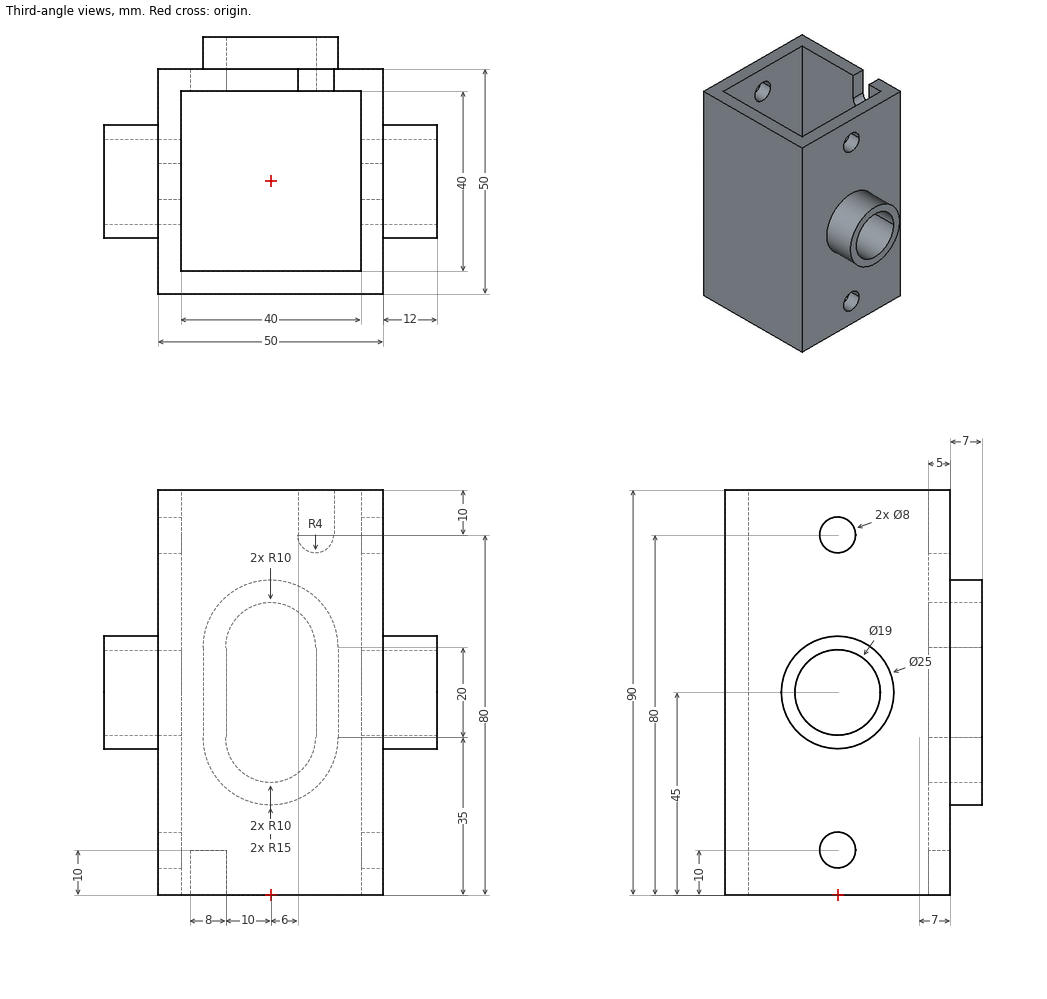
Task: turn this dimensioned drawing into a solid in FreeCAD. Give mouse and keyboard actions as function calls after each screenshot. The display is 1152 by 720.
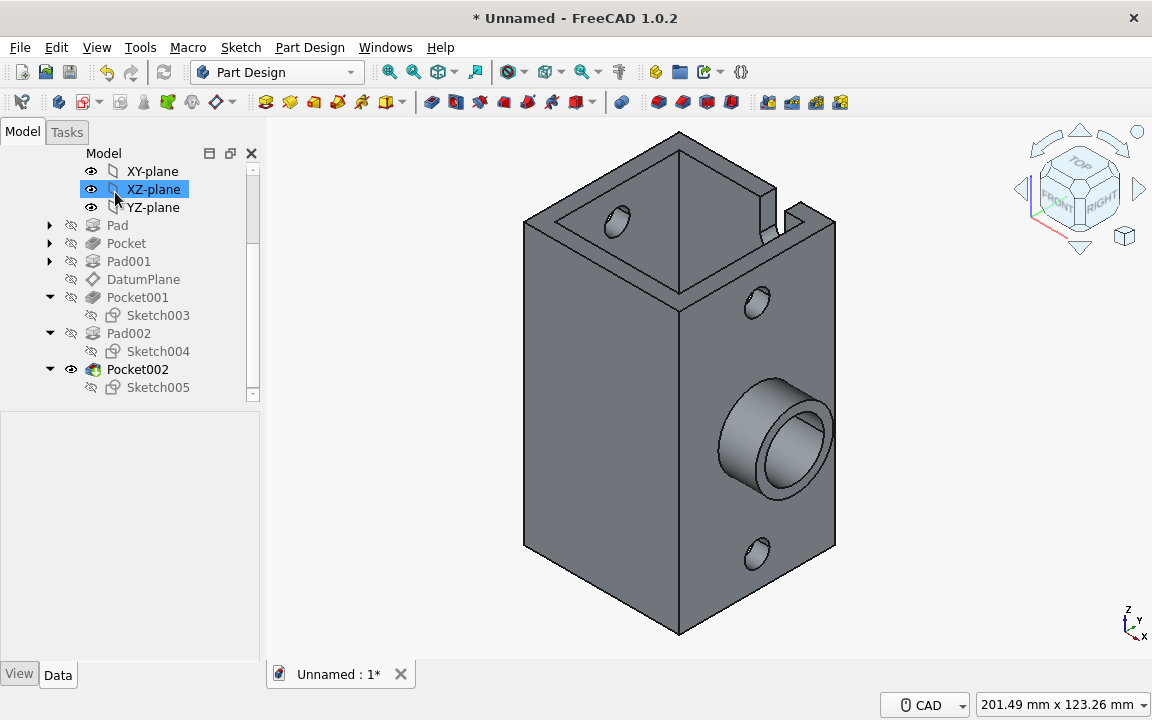
click(116, 333)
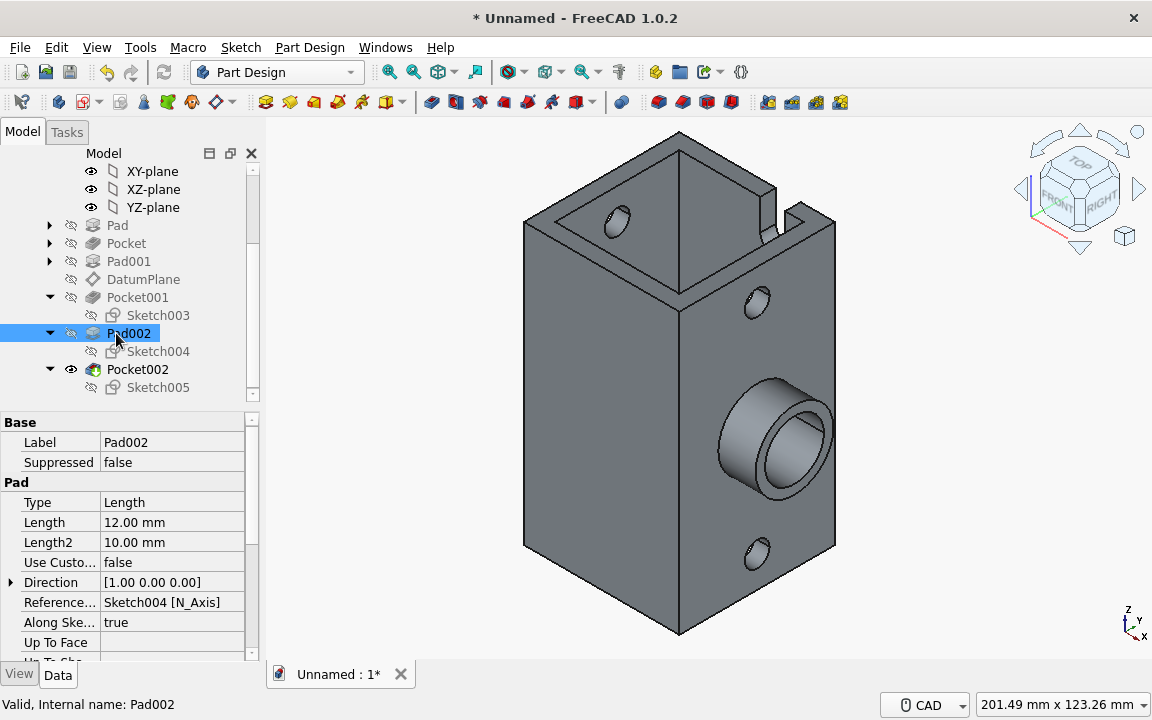
click(768, 102)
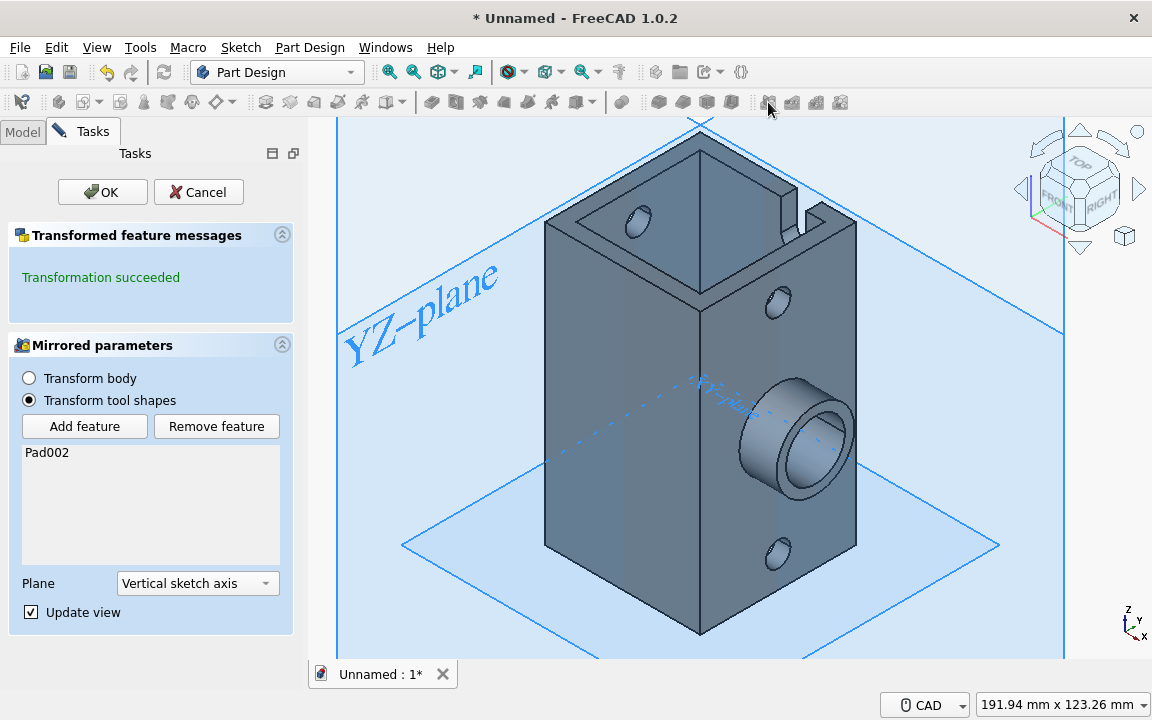
click(198, 584)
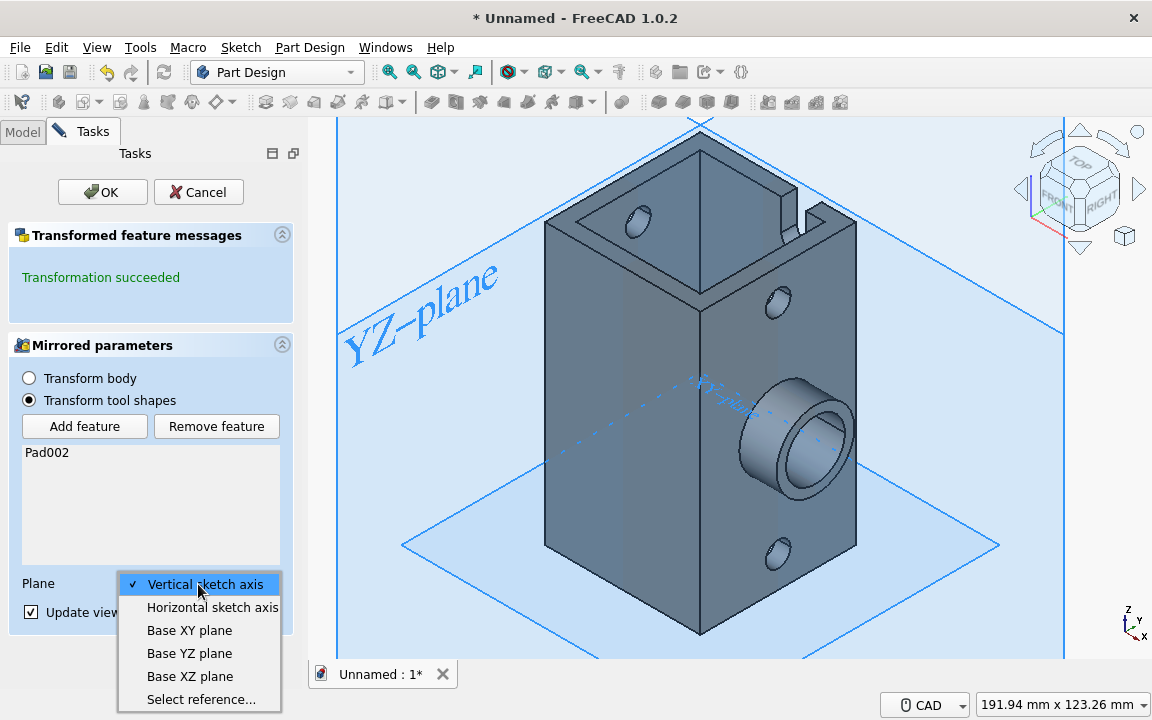
click(198, 654)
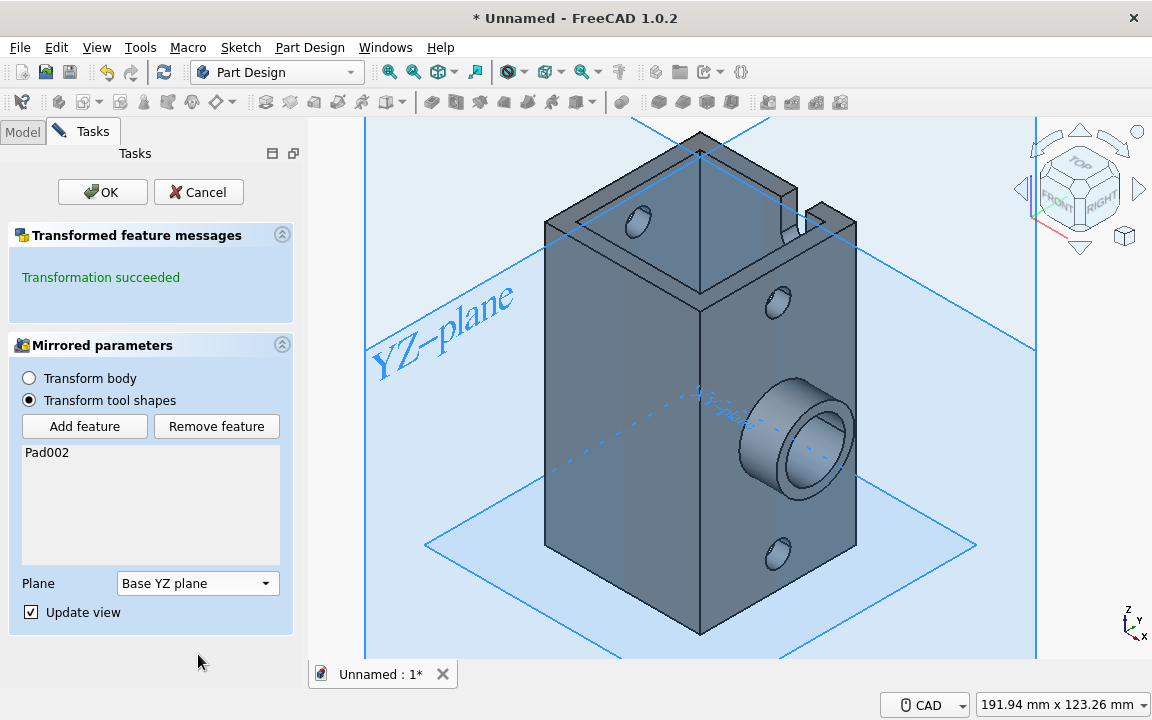
click(103, 192)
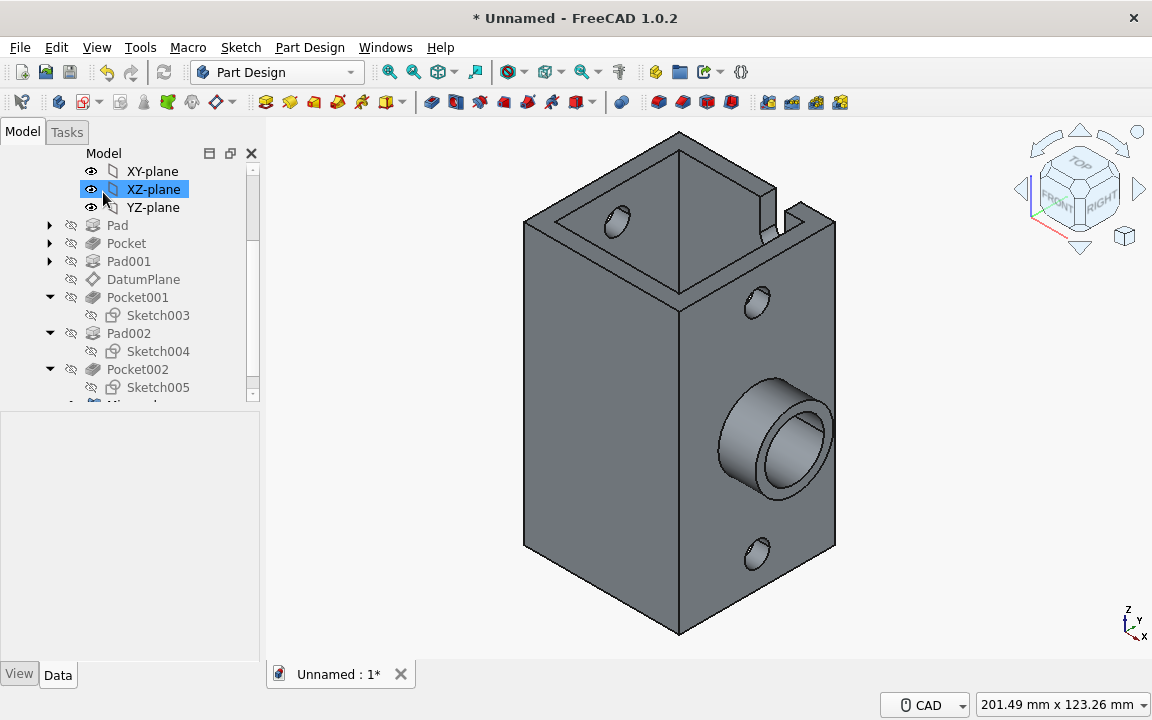
key(v)
key(f)